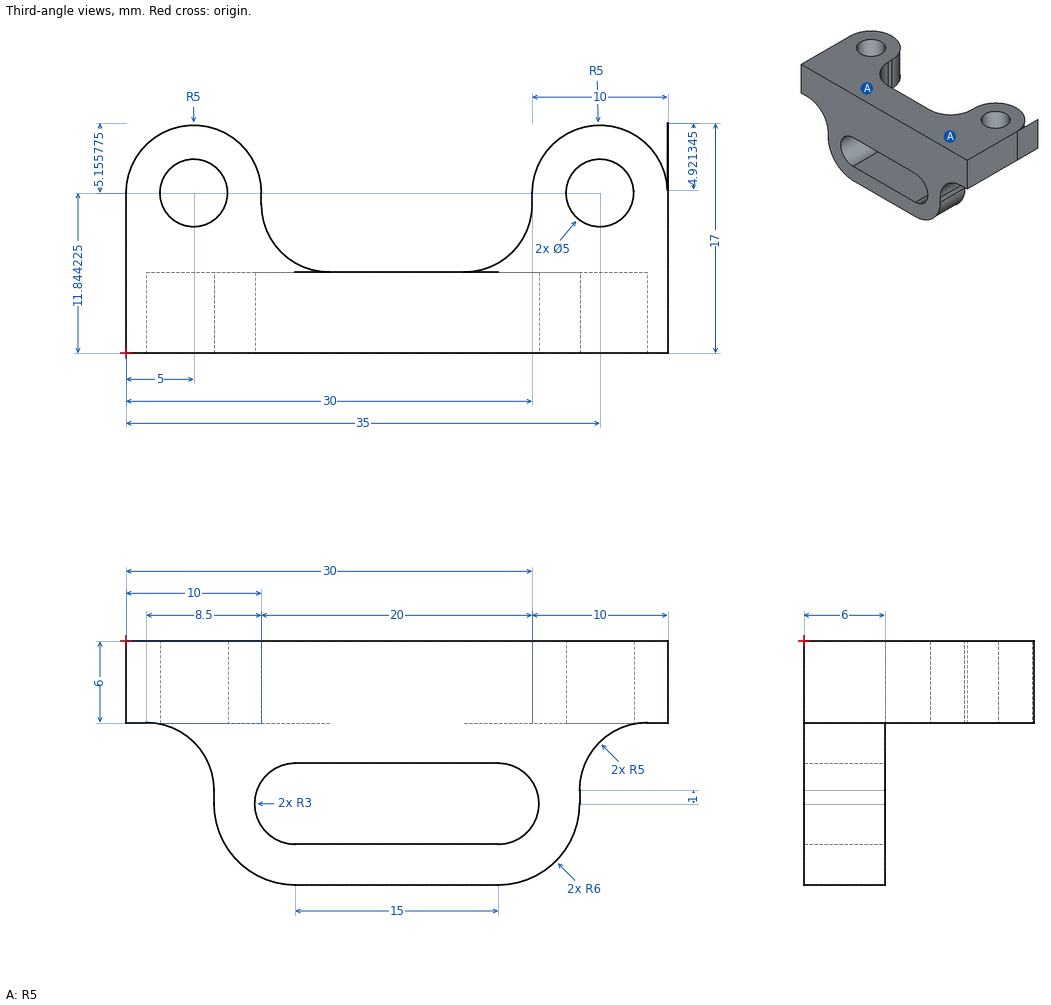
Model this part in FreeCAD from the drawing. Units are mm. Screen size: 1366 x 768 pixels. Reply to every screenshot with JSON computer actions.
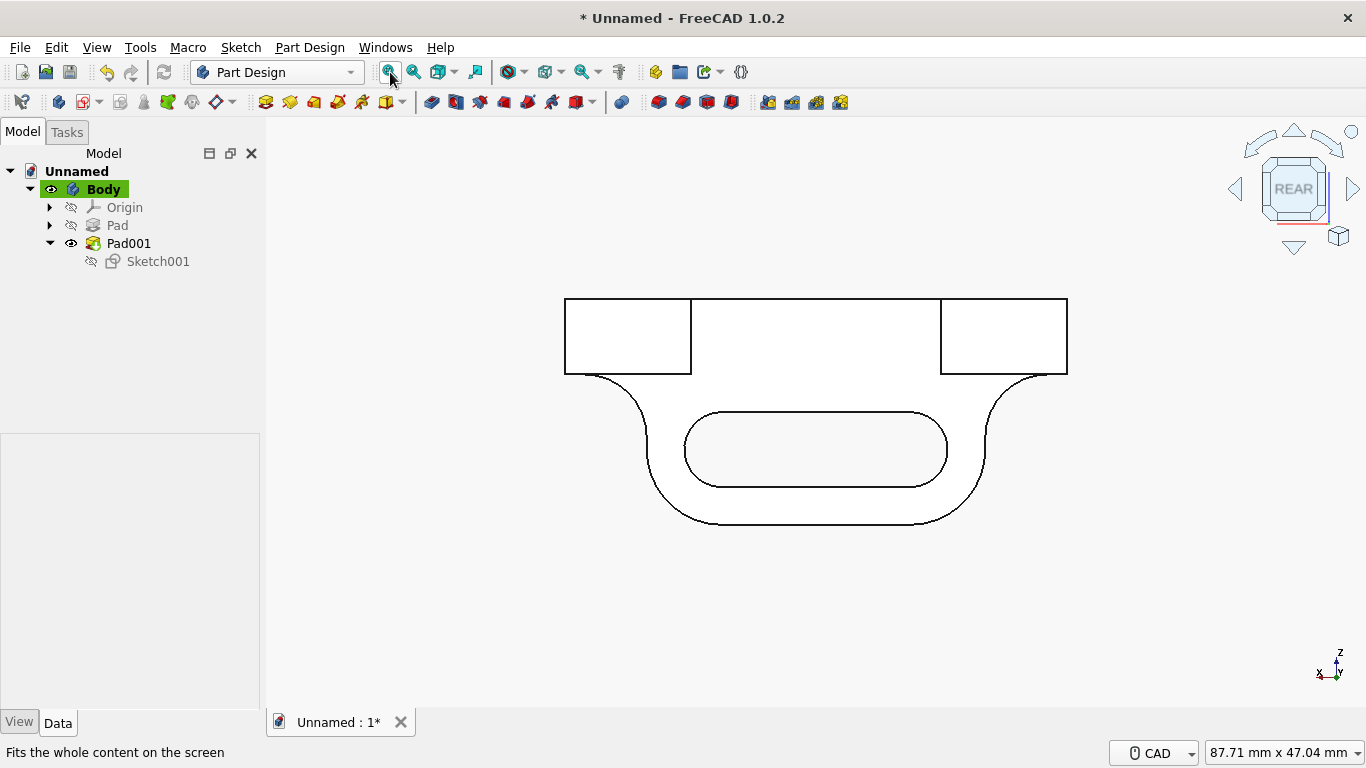
{"action": "key", "text": "6"}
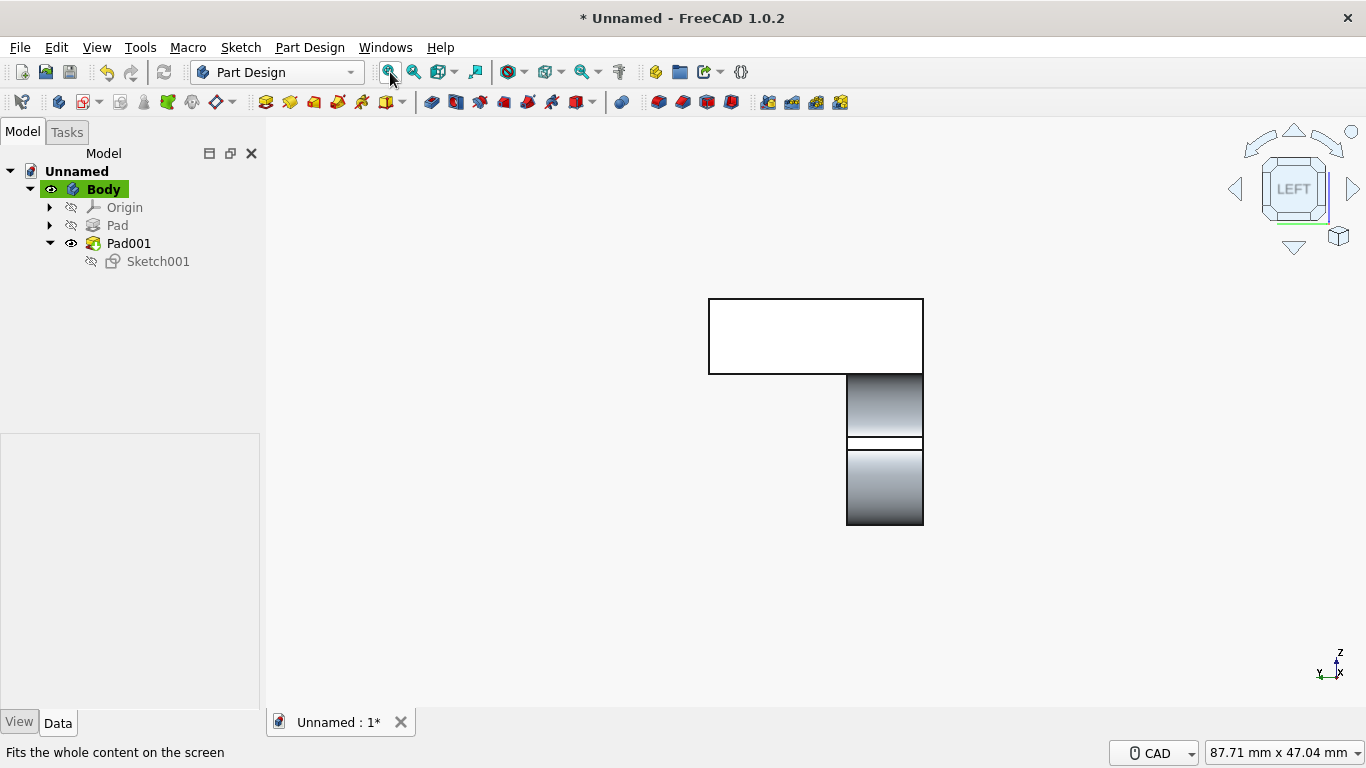
{"action": "left_click", "coordinate": [390, 72]}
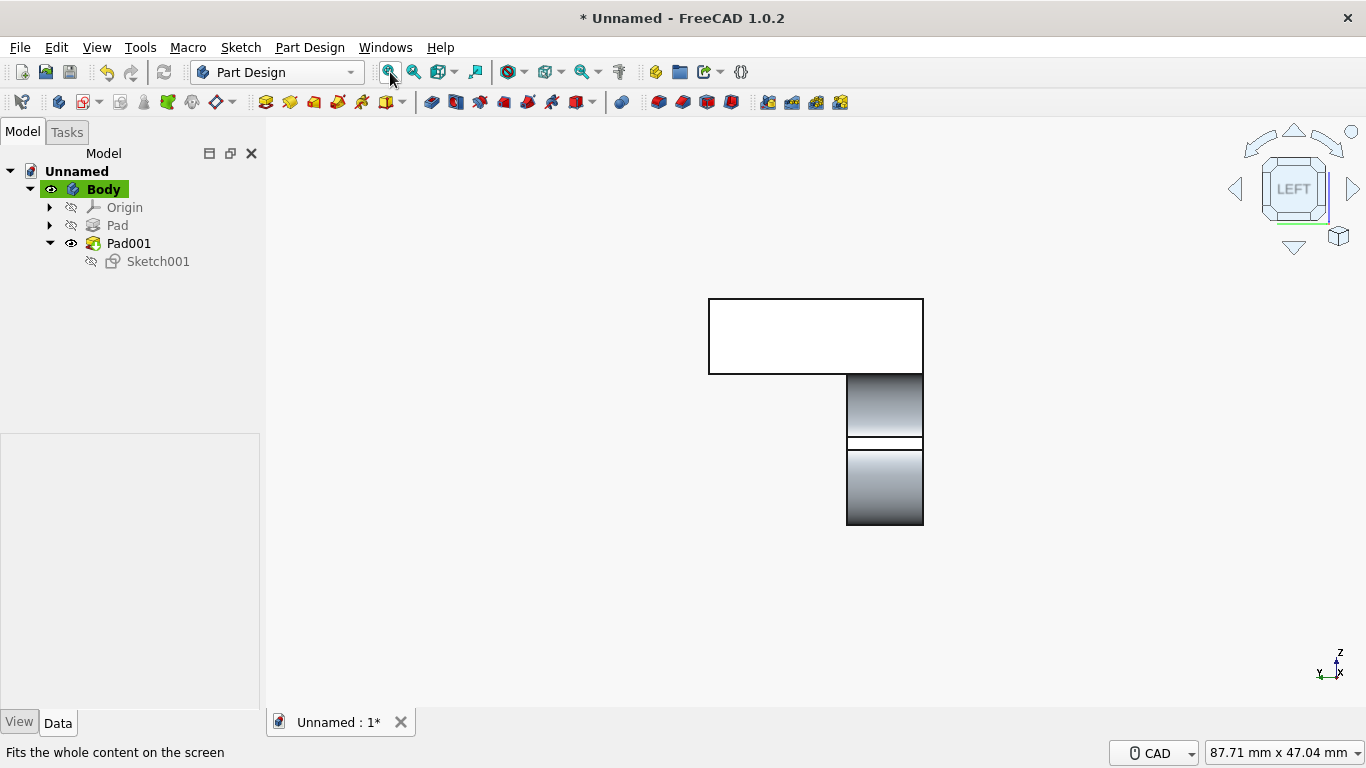
{"action": "key", "text": "v 3"}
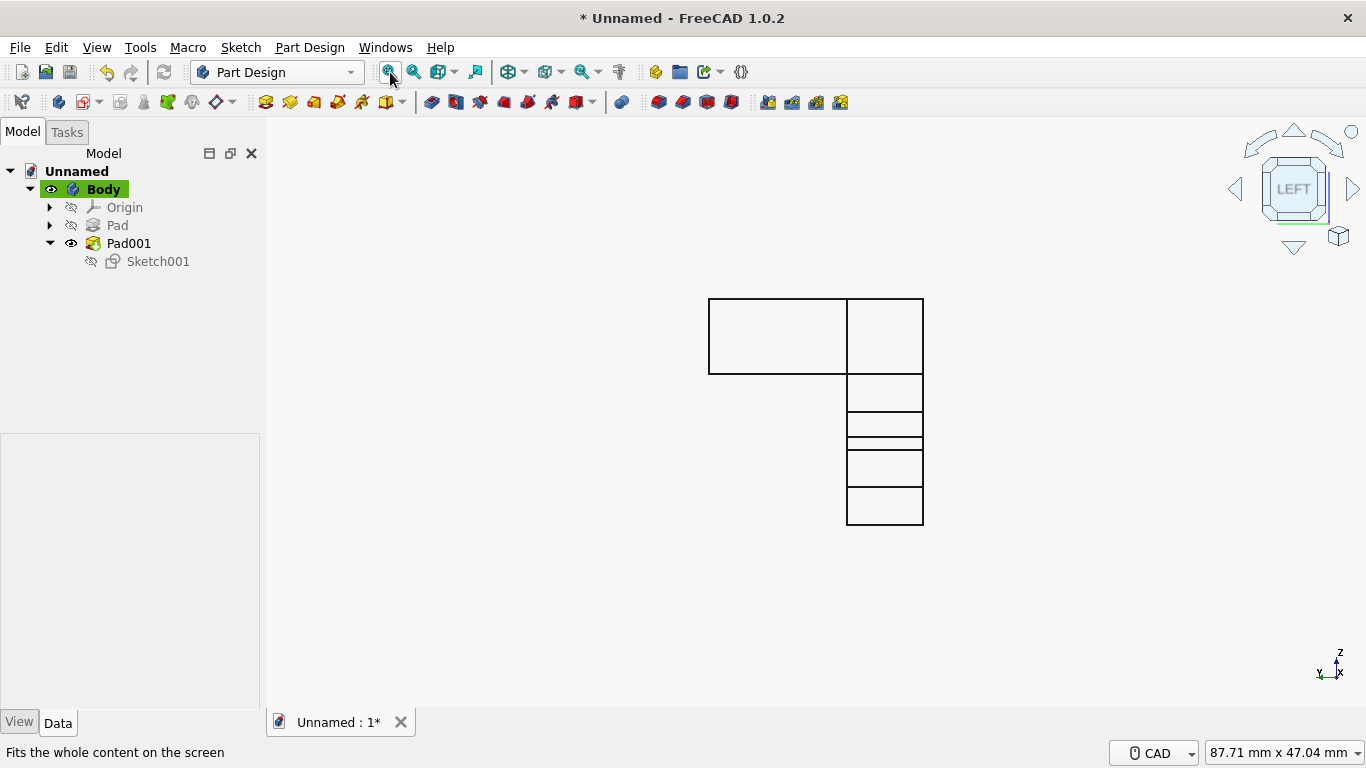
{"action": "key", "text": "0"}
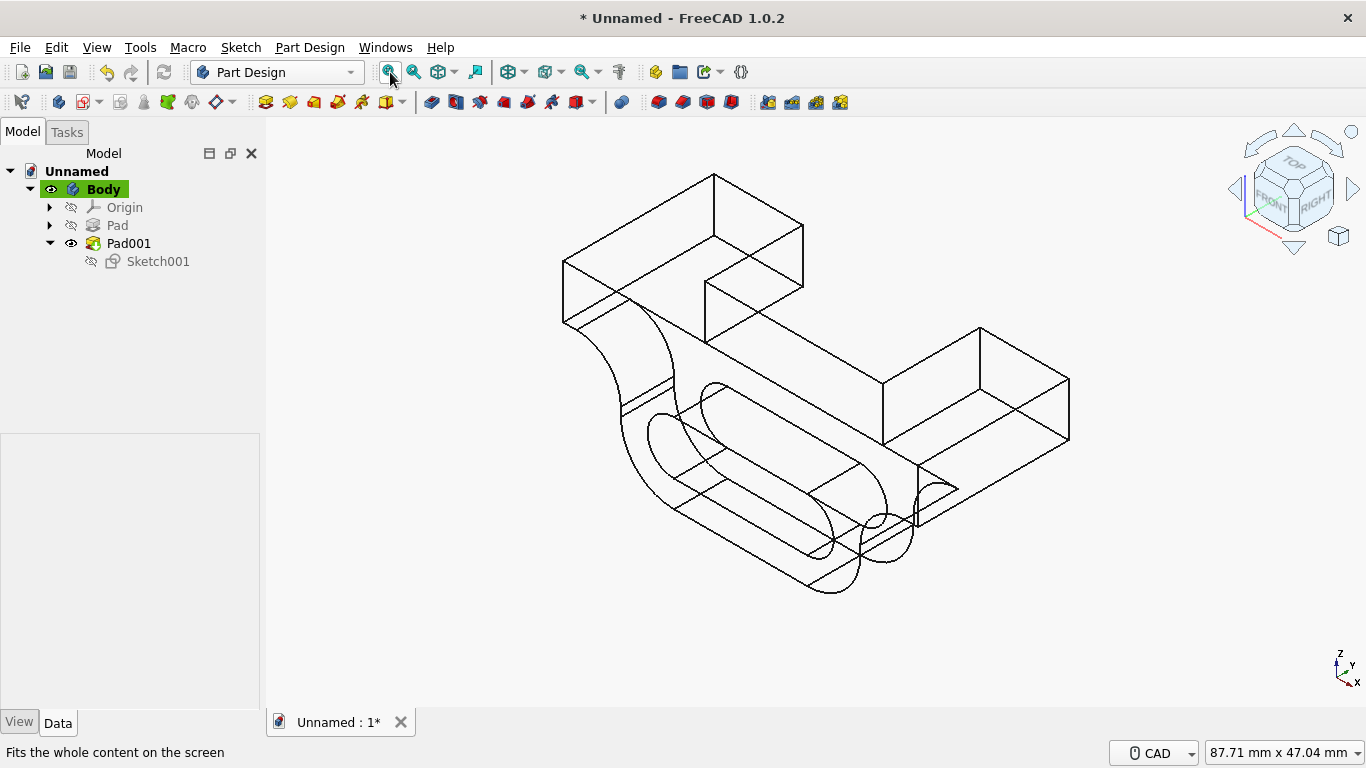
{"action": "left_click", "coordinate": [705, 311]}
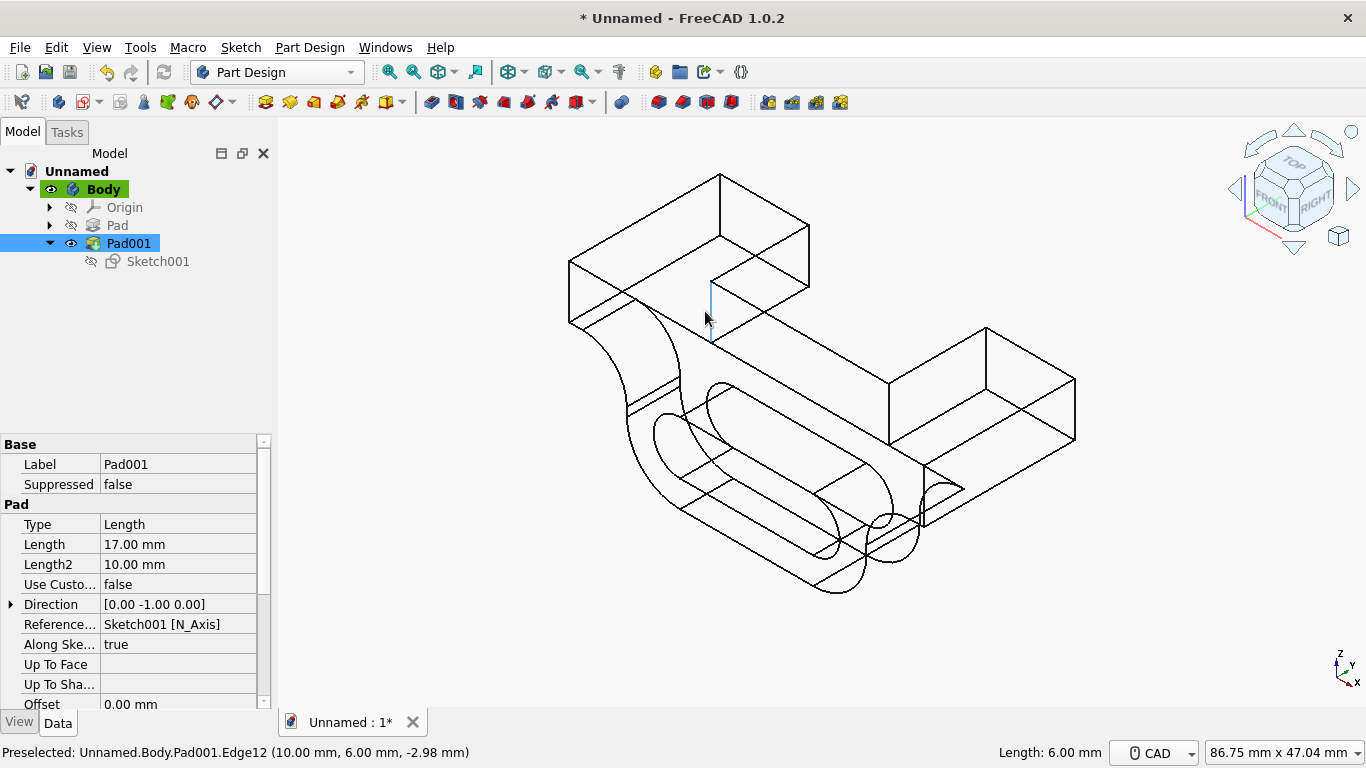
{"action": "left_click", "coordinate": [889, 414], "text": "ctrl"}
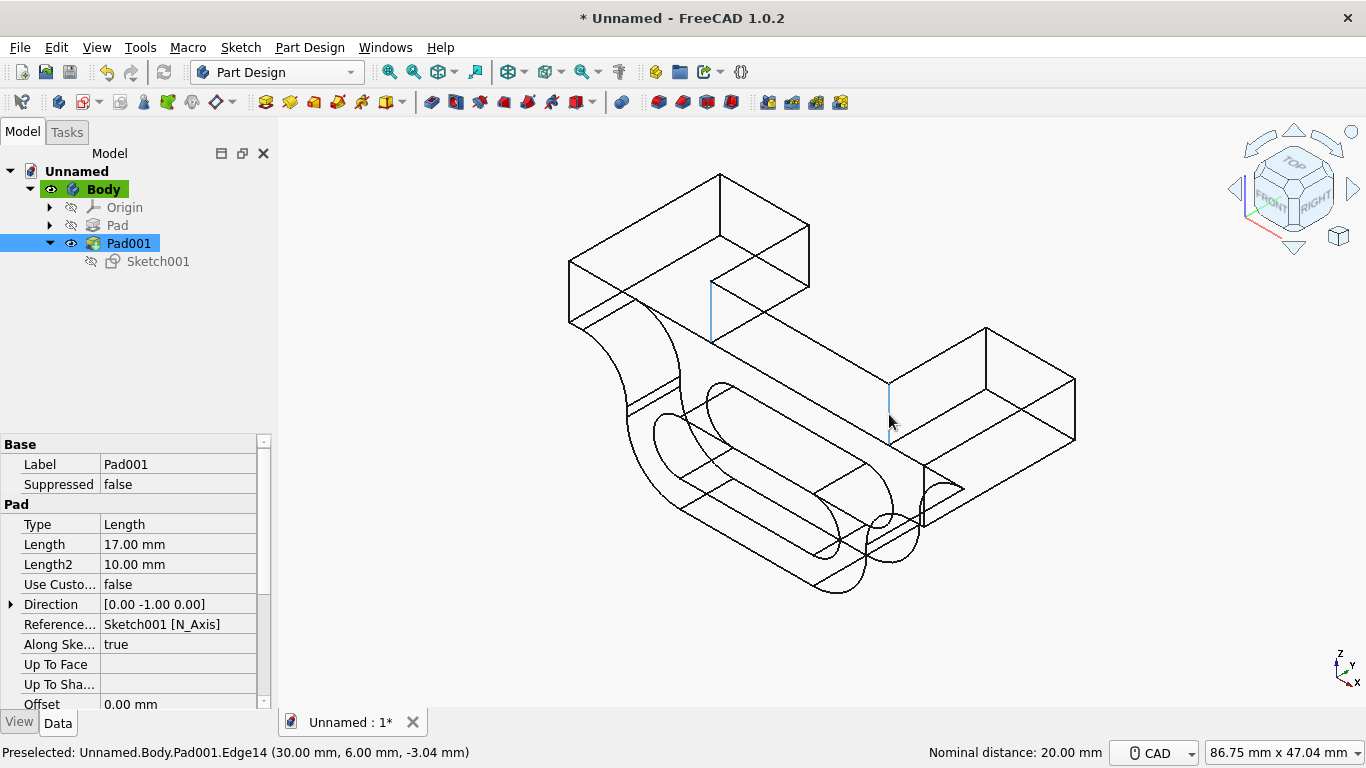
{"action": "key", "text": "v 1"}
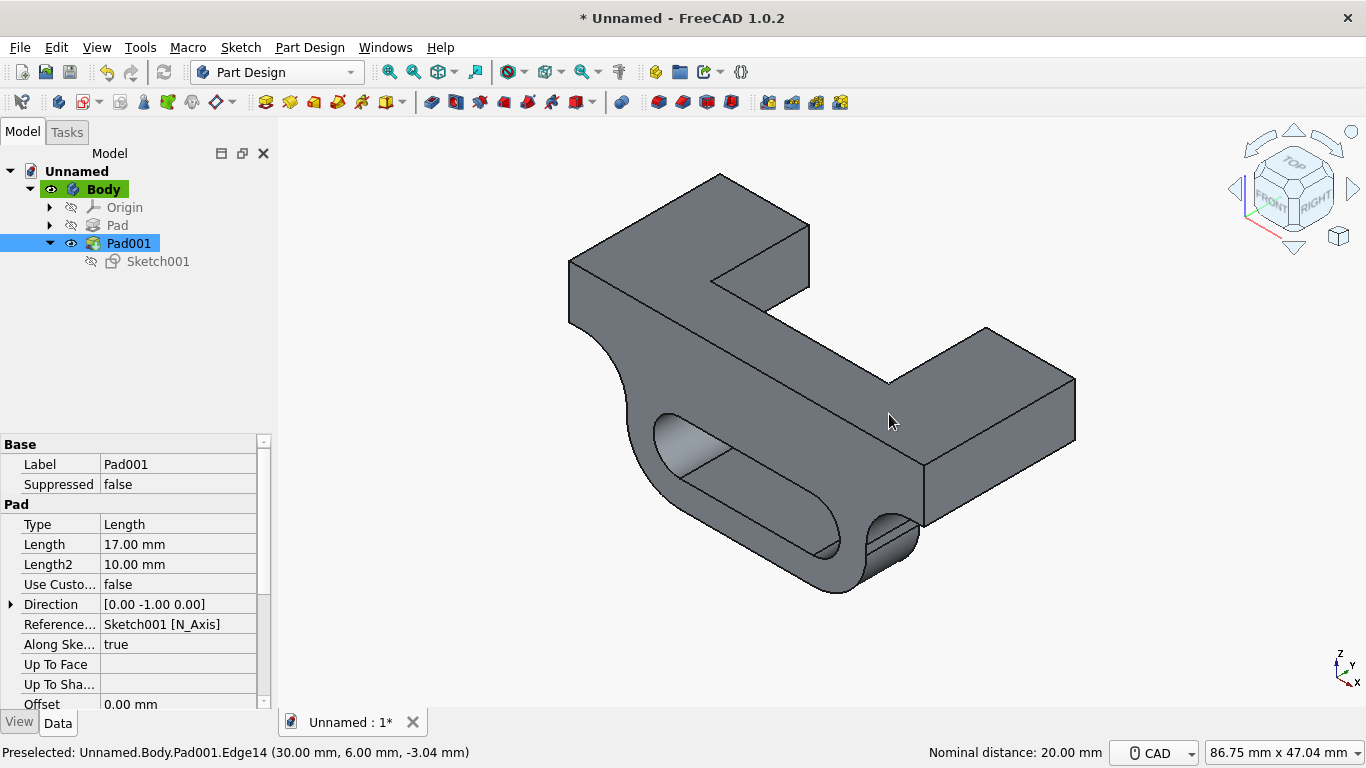
{"action": "left_click", "coordinate": [660, 102]}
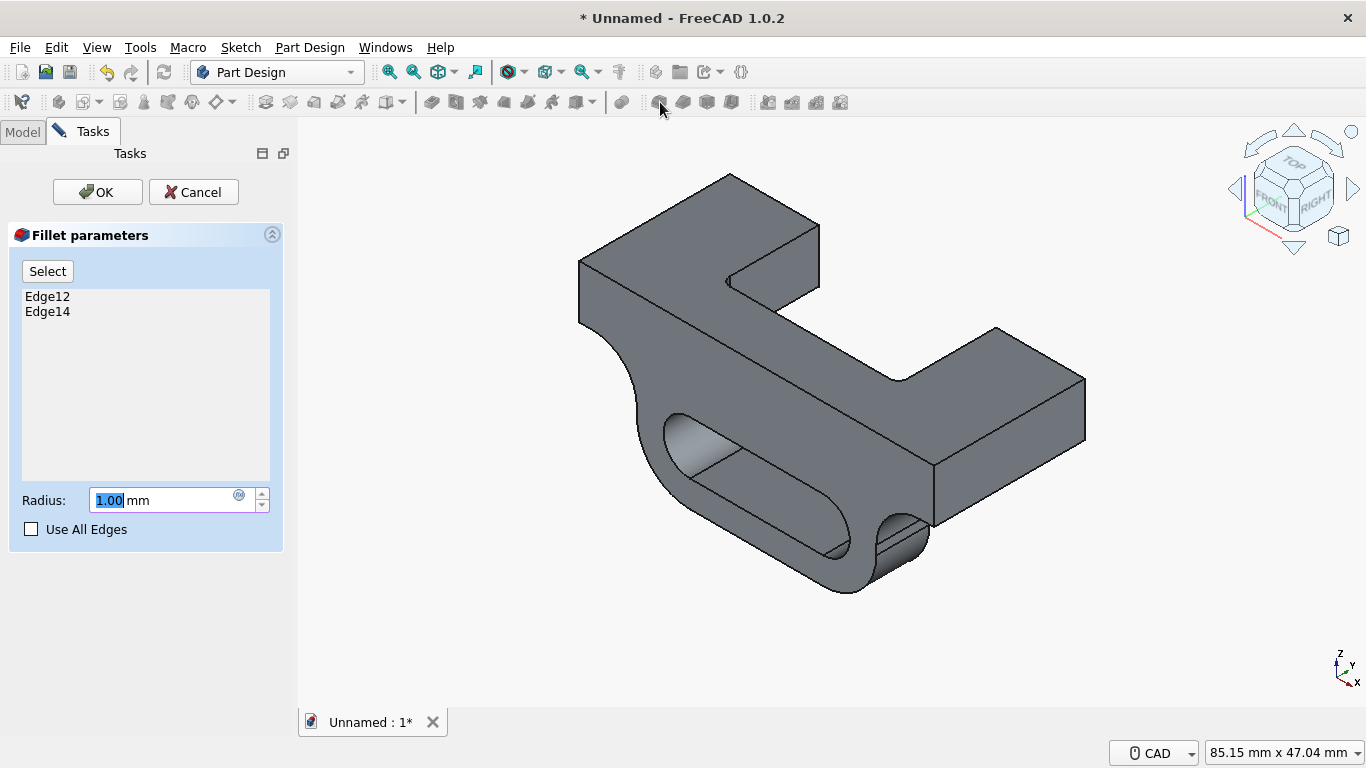
{"action": "type", "text": "5"}
{"action": "key", "text": "Tab"}